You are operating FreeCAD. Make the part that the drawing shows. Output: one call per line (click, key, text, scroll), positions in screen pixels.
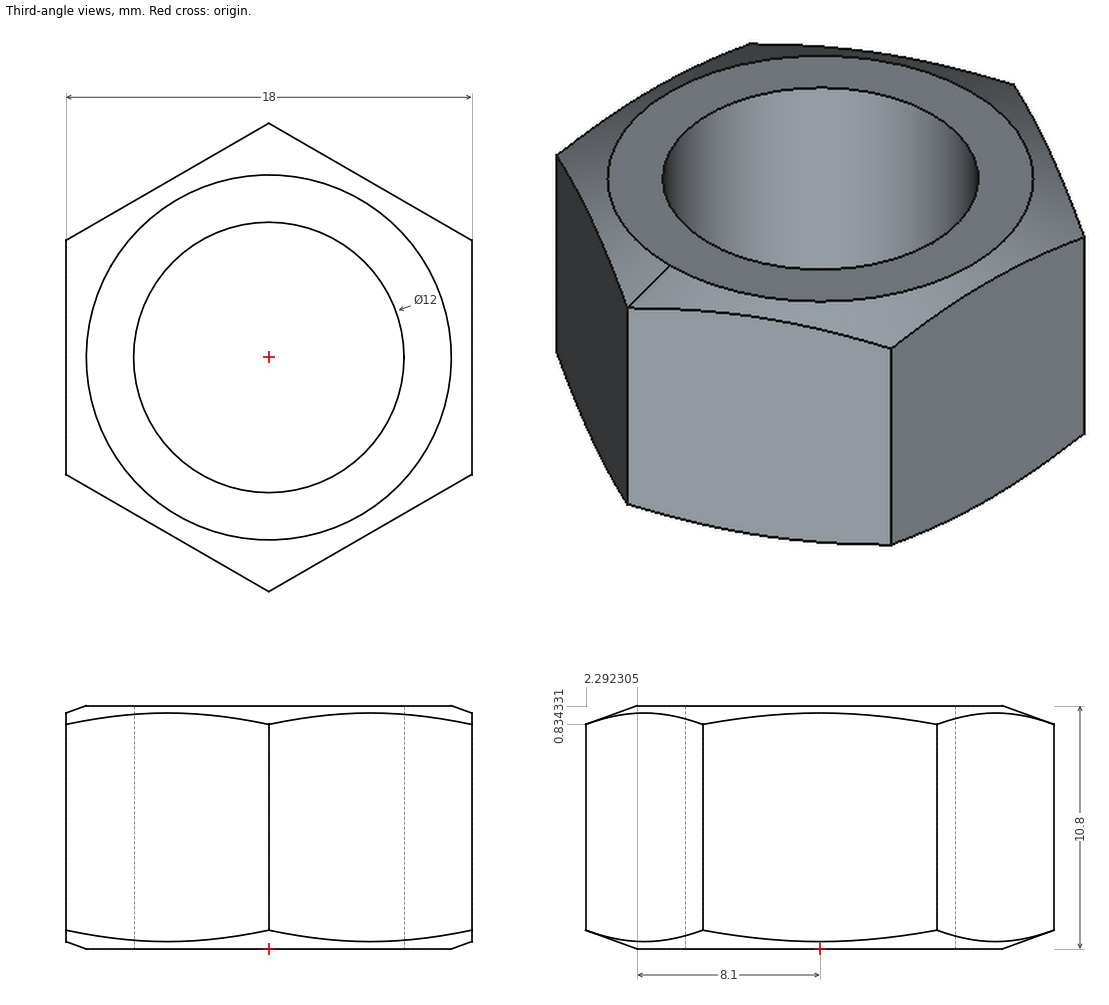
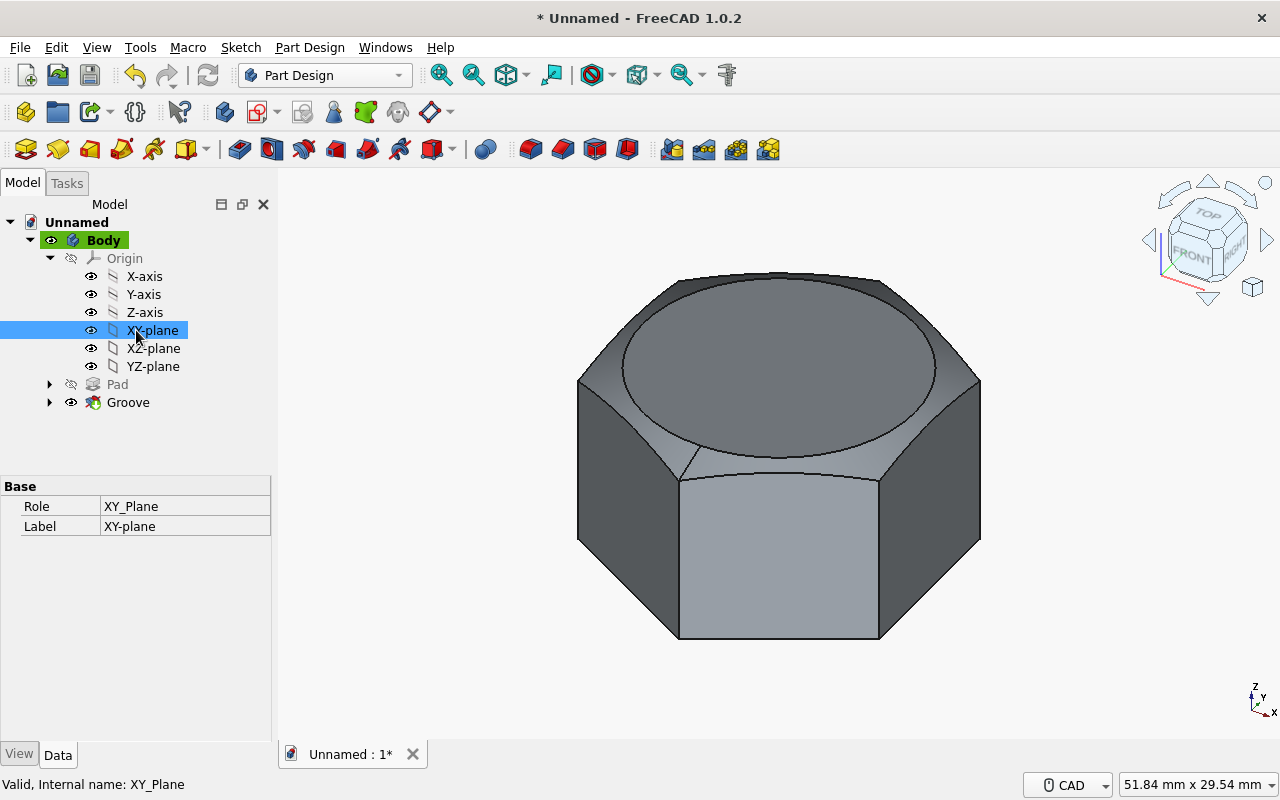
click(430, 112)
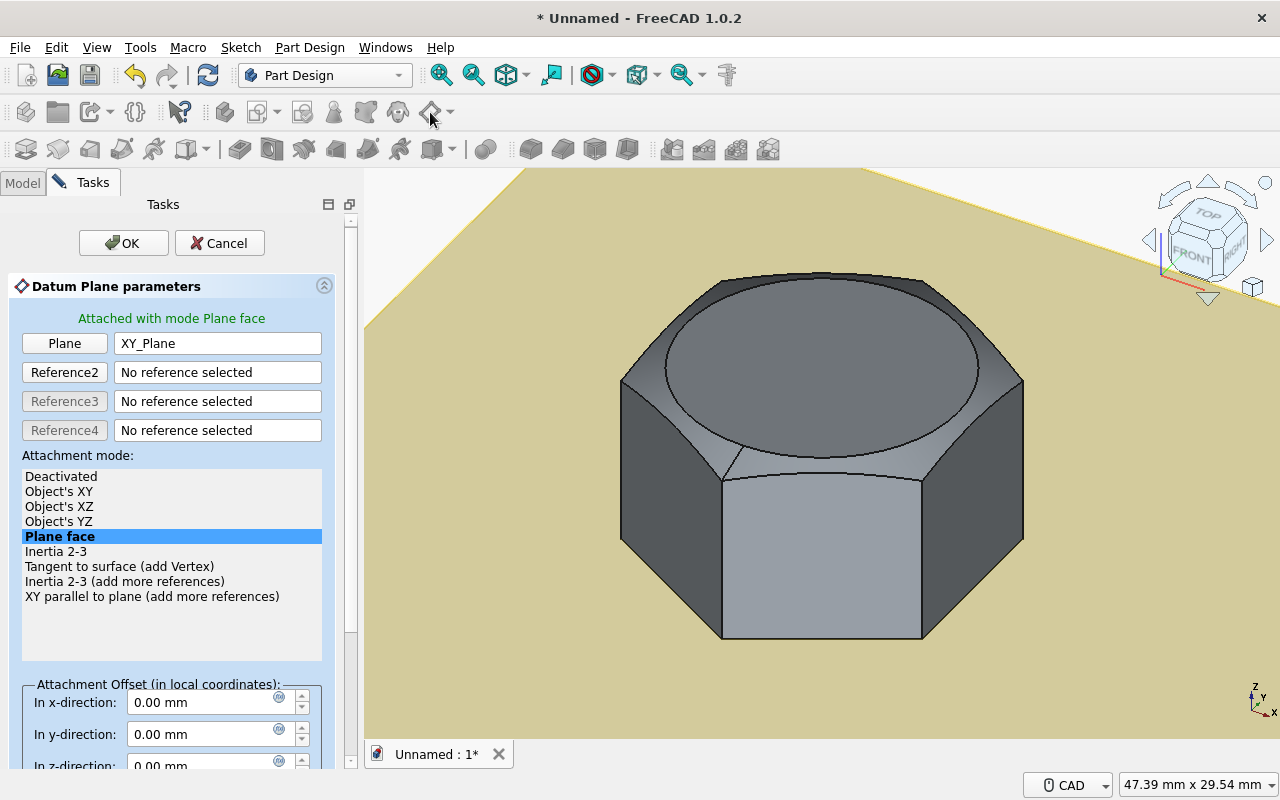
scroll(351, 491, down, 2)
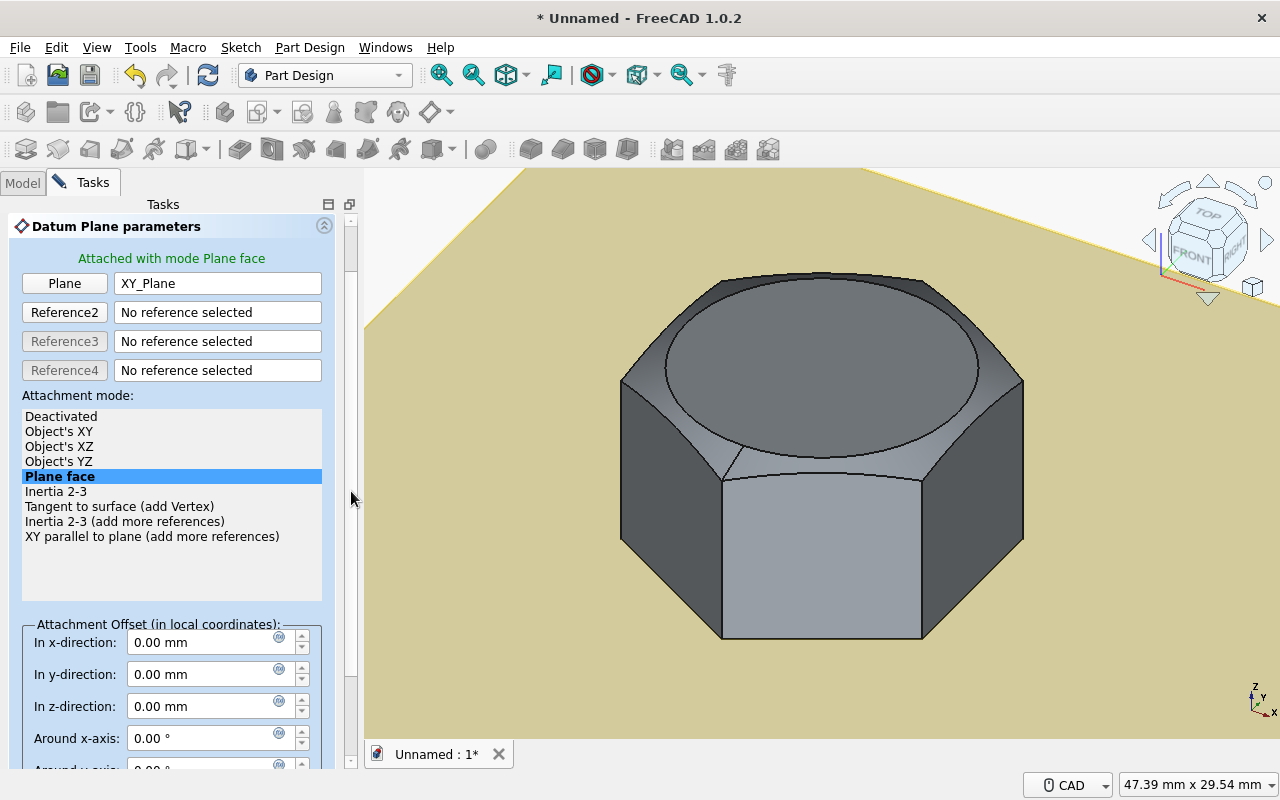
triple_click(210, 646)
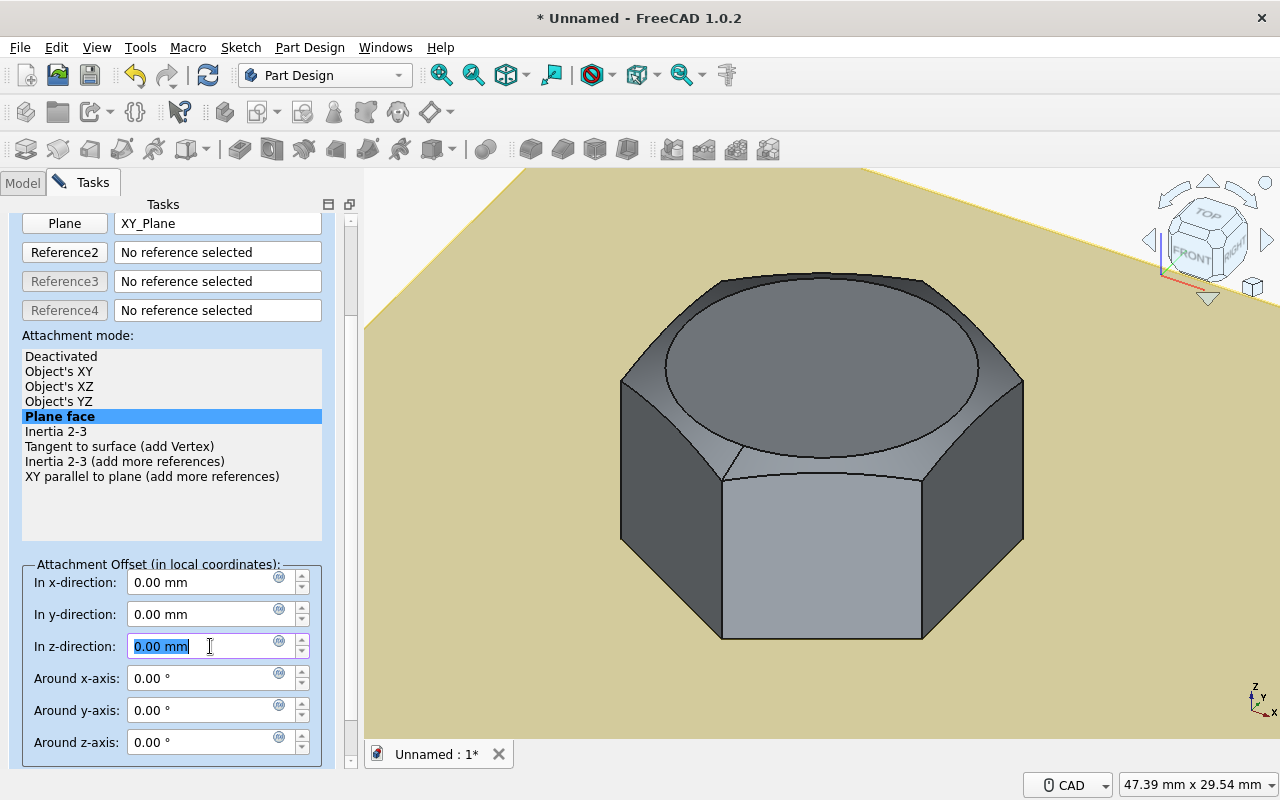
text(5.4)
key(Tab)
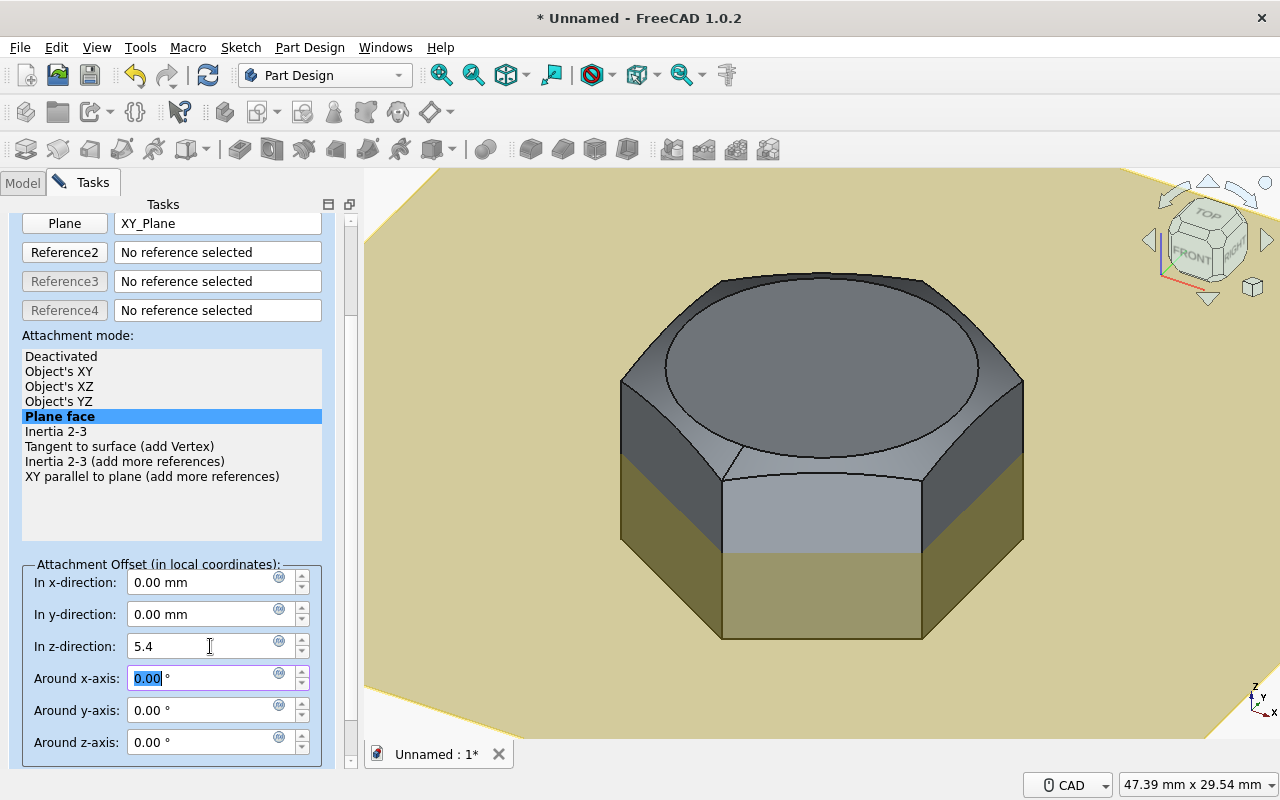
scroll(351, 491, up, 3)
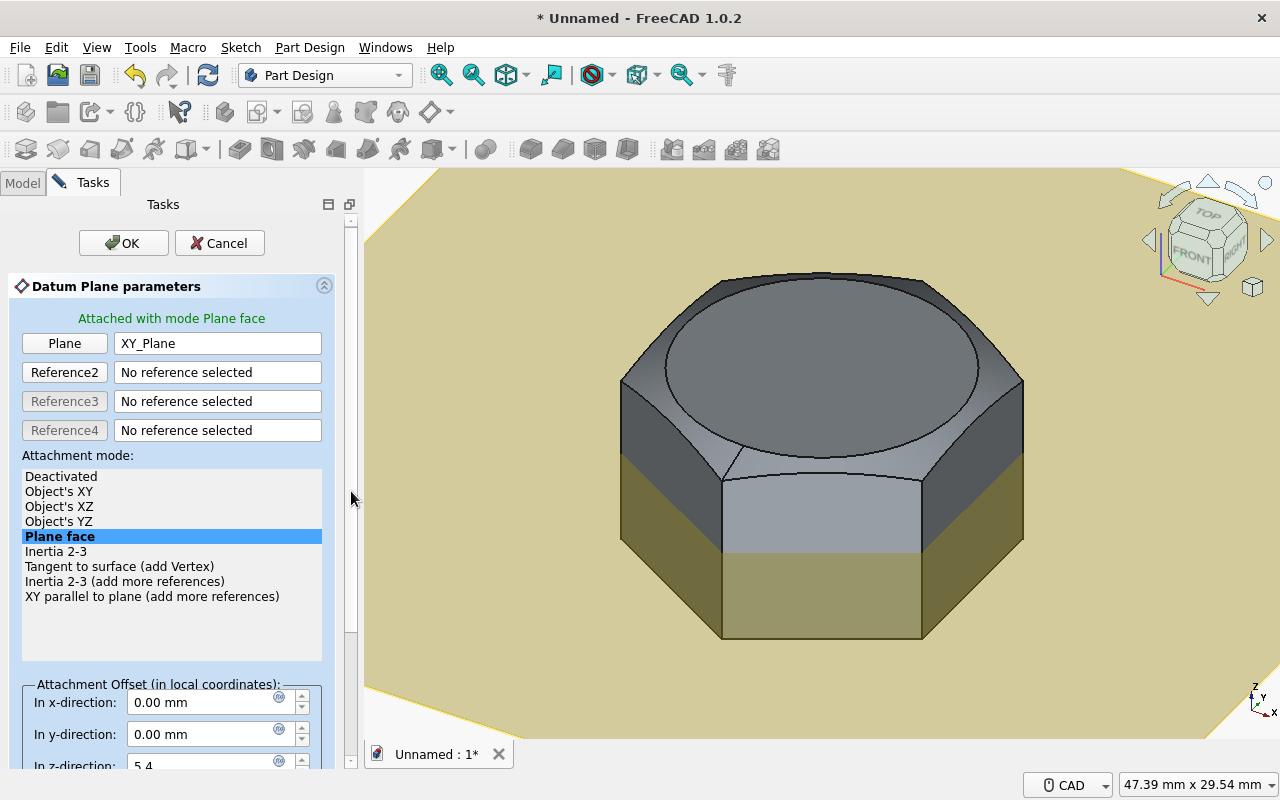
click(124, 243)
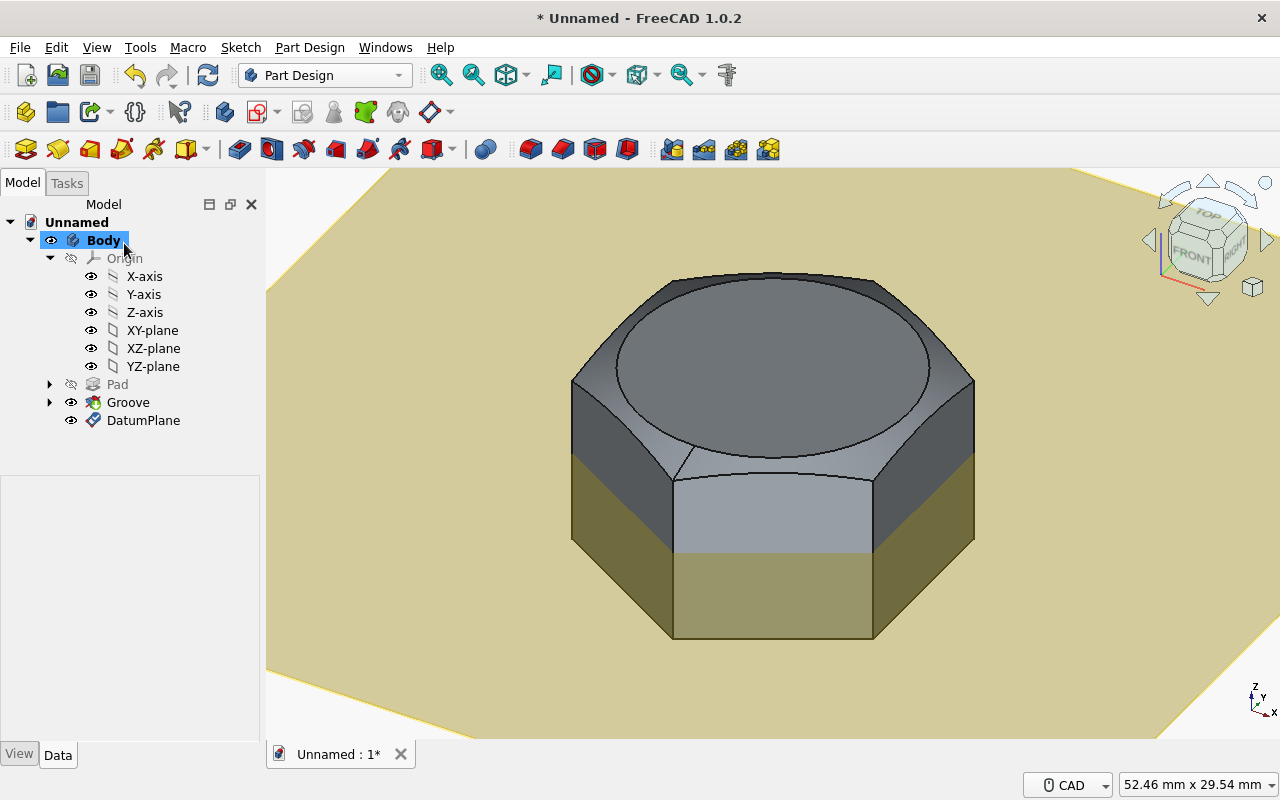
click(116, 402)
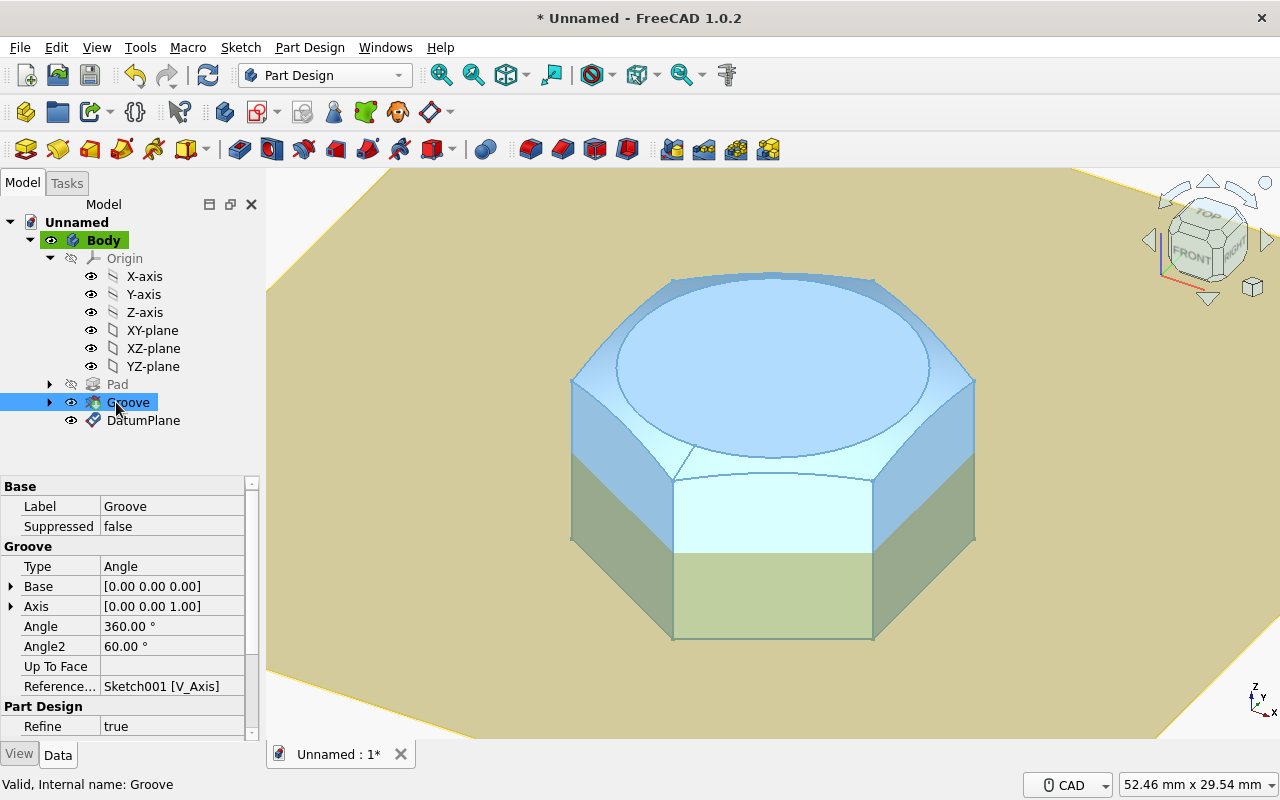
click(672, 150)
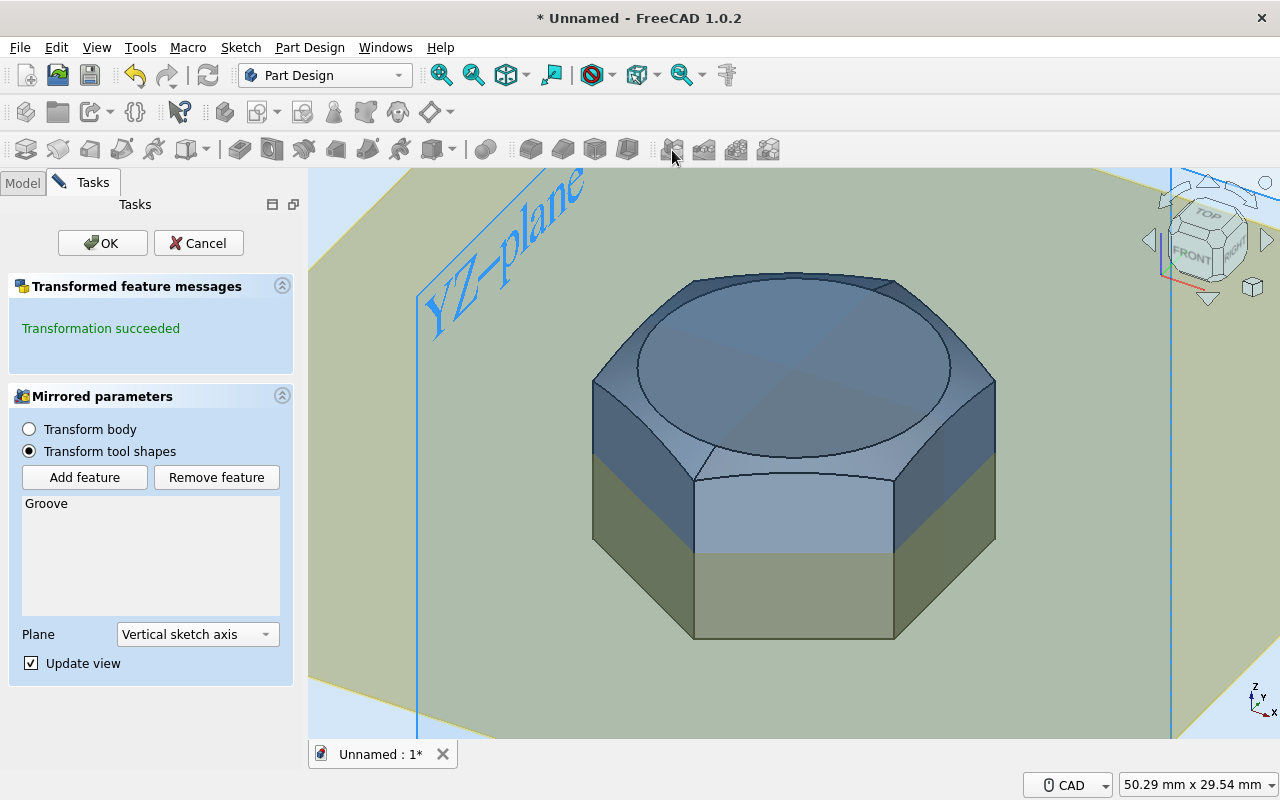
click(198, 634)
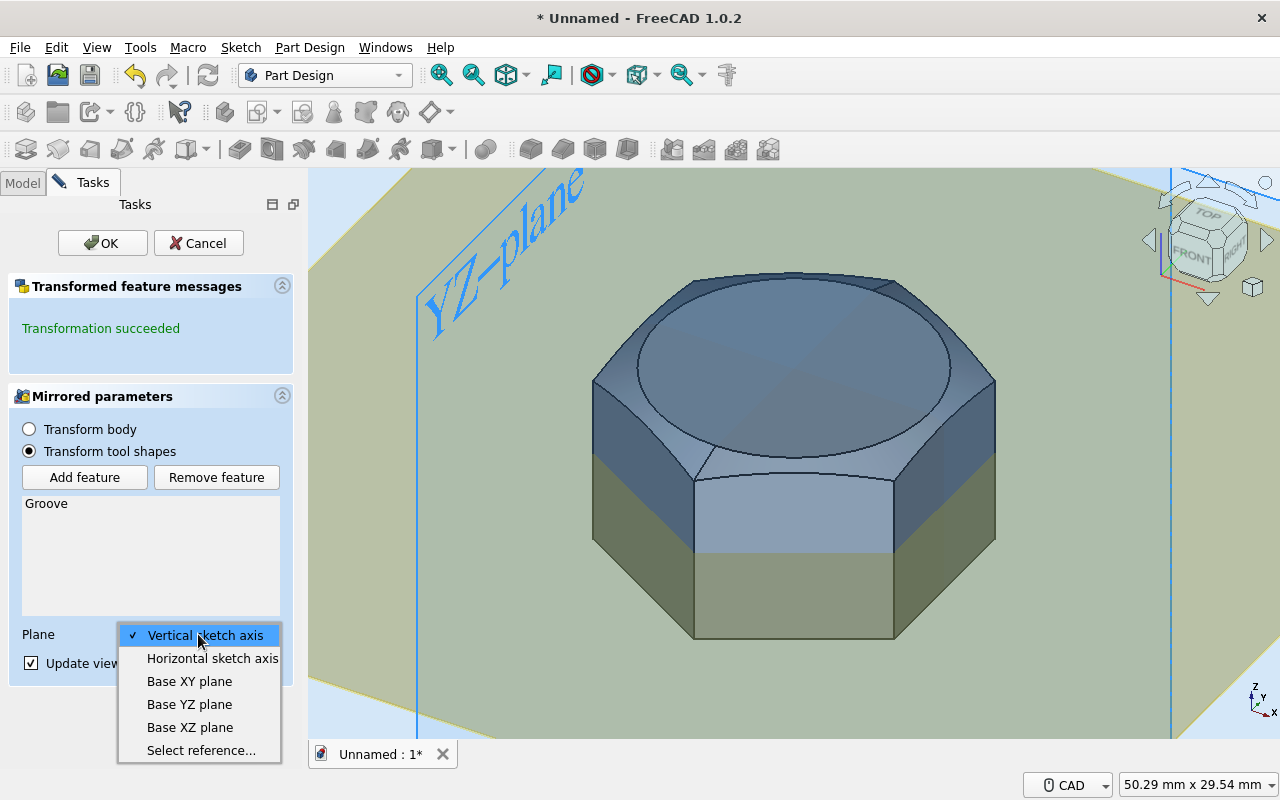
click(198, 750)